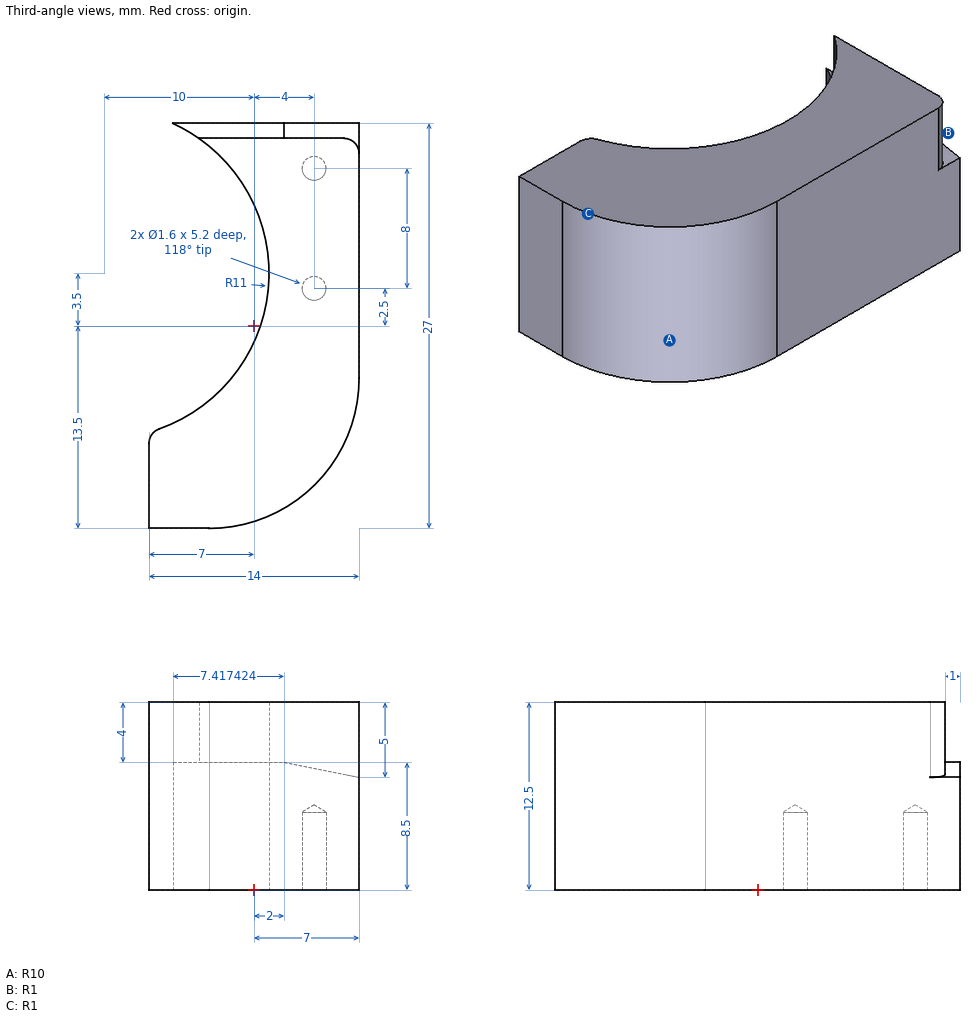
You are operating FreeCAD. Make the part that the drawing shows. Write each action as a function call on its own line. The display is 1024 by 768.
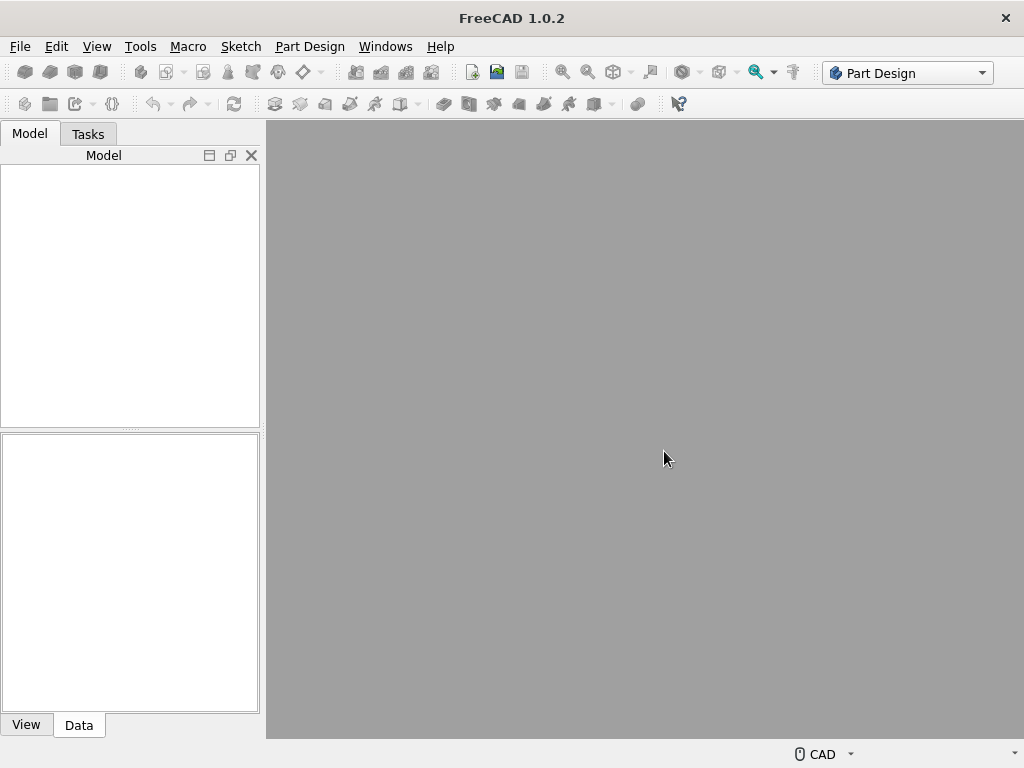
click(472, 72)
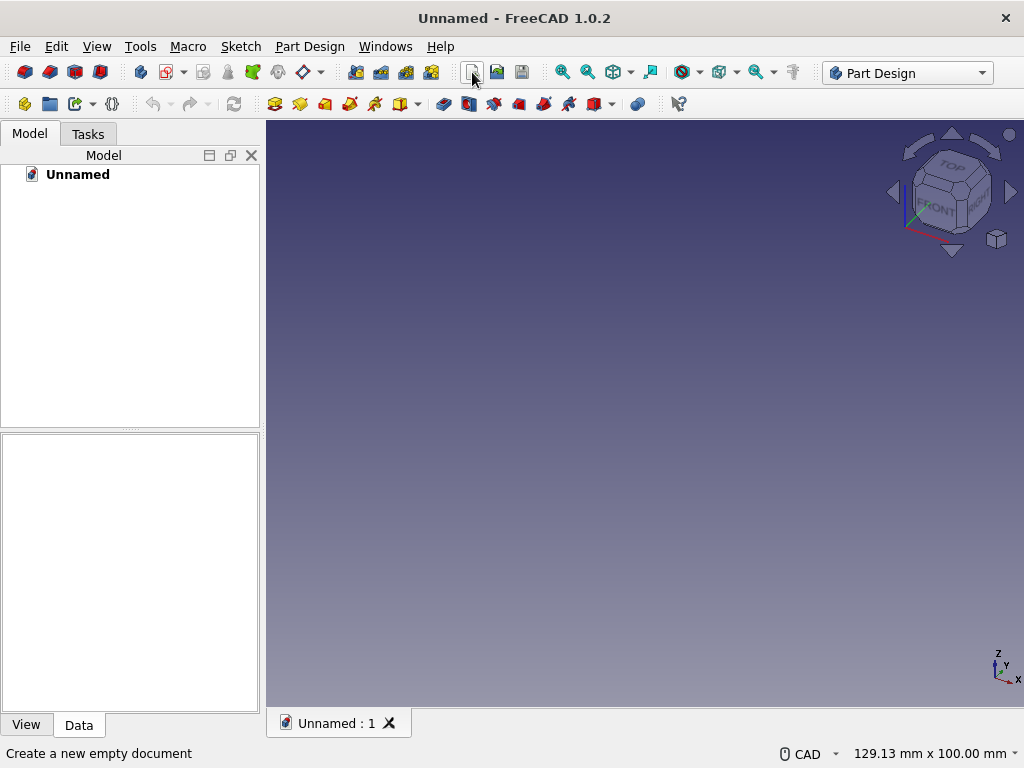
click(166, 72)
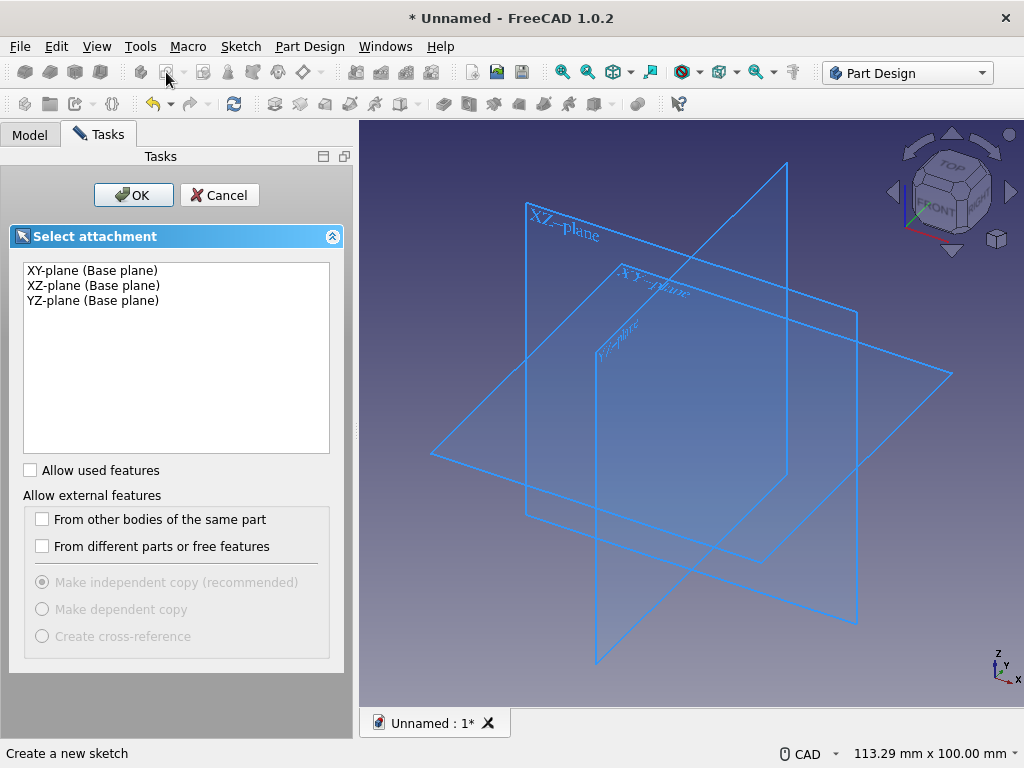
click(84, 270)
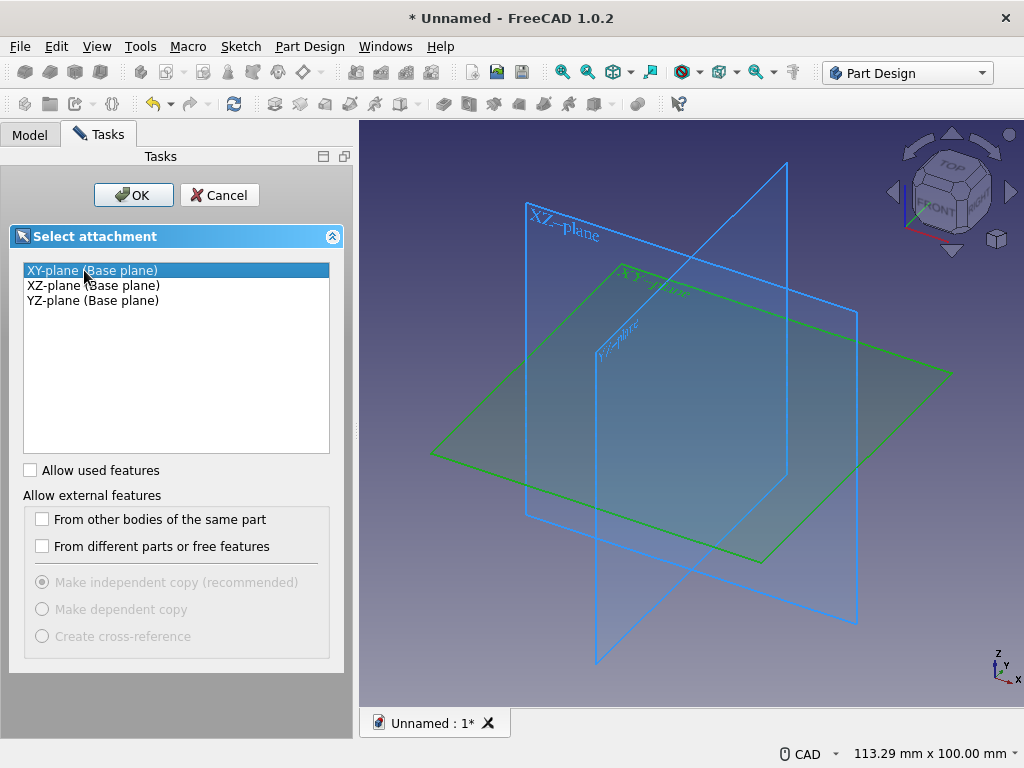
click(134, 195)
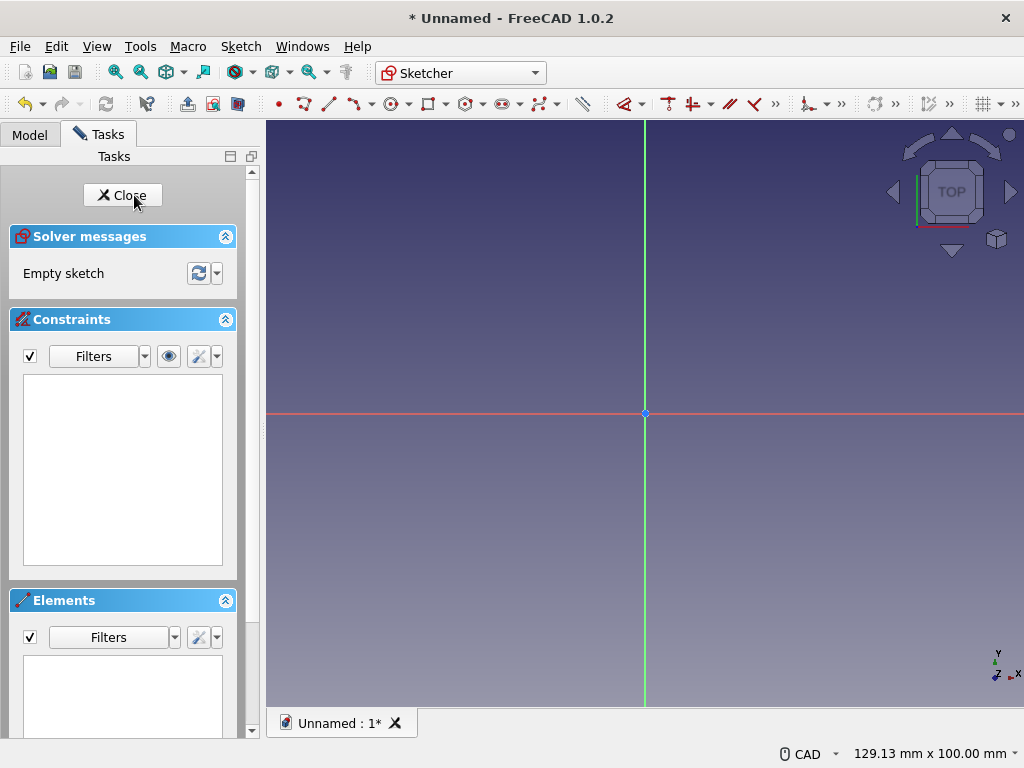
scroll(701, 413, up, 4)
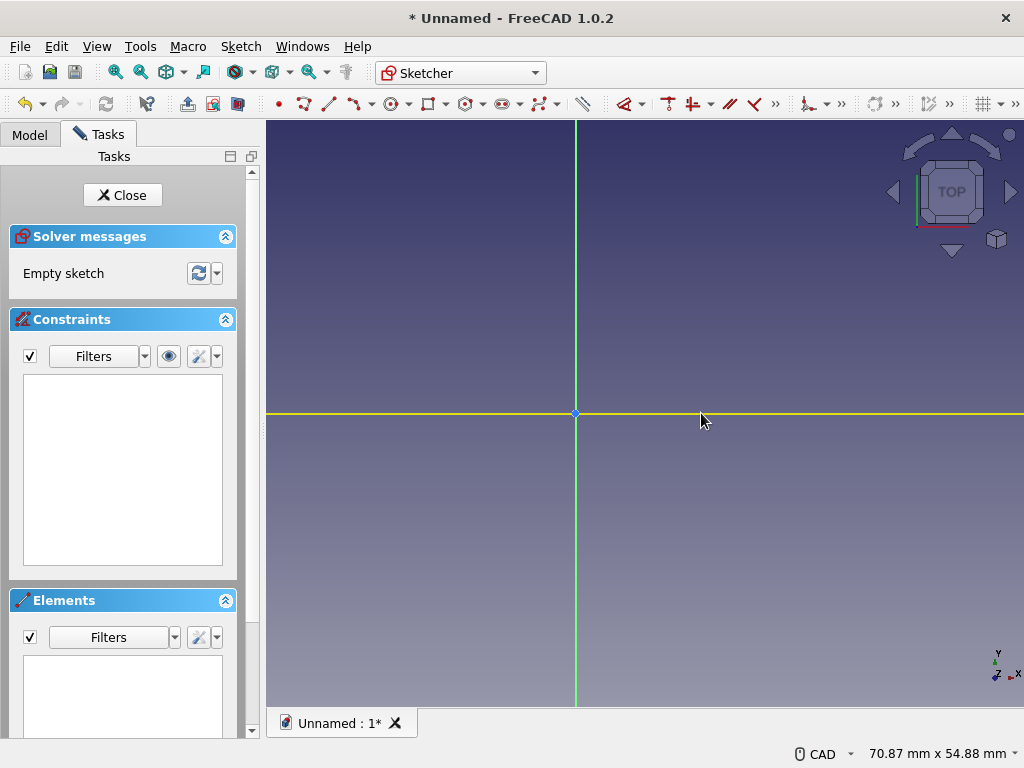
click(304, 104)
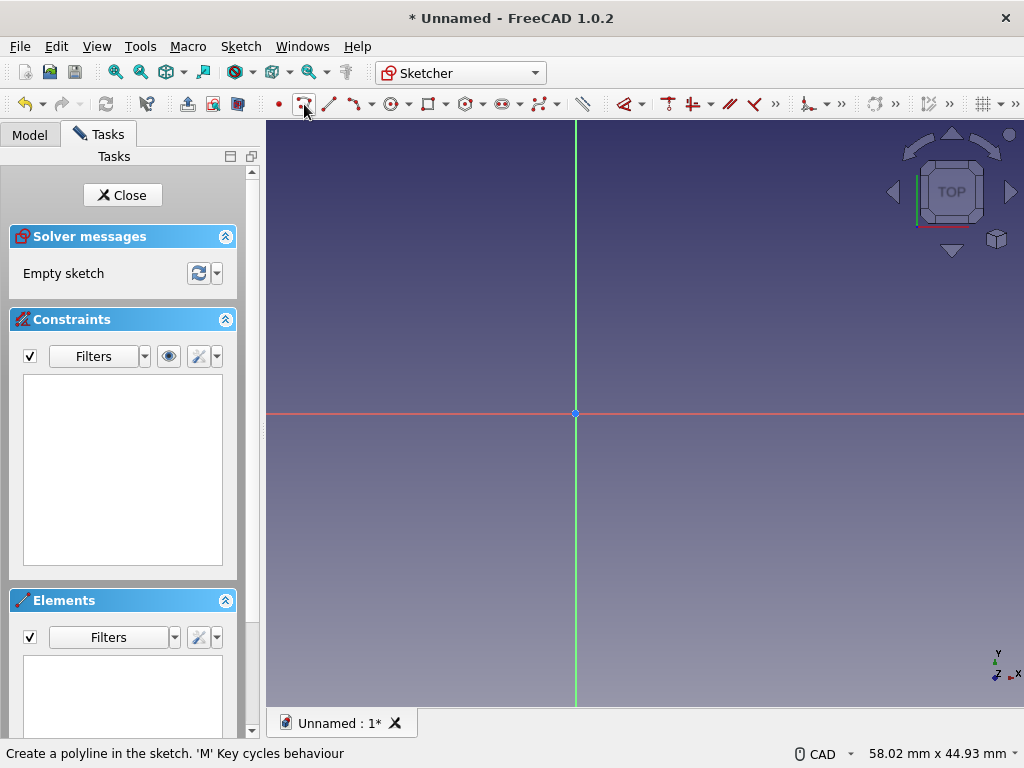
click(484, 506)
click(484, 590)
click(667, 590)
click(667, 237)
click(505, 237)
right_click(505, 237)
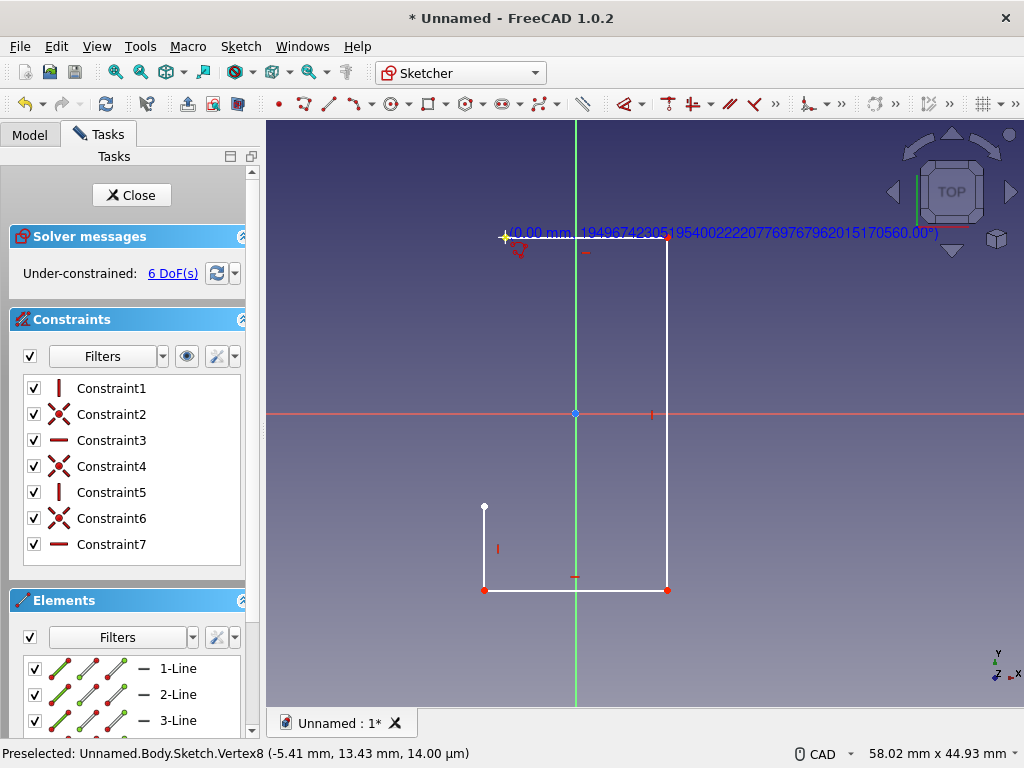
click(354, 104)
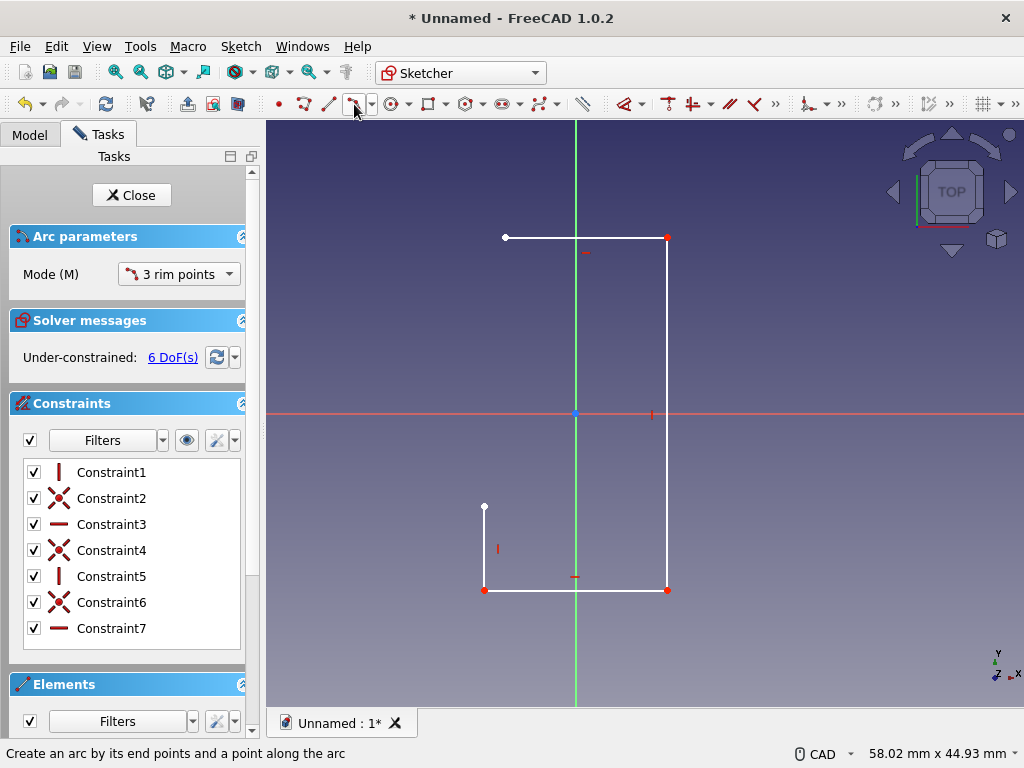
click(505, 238)
click(484, 507)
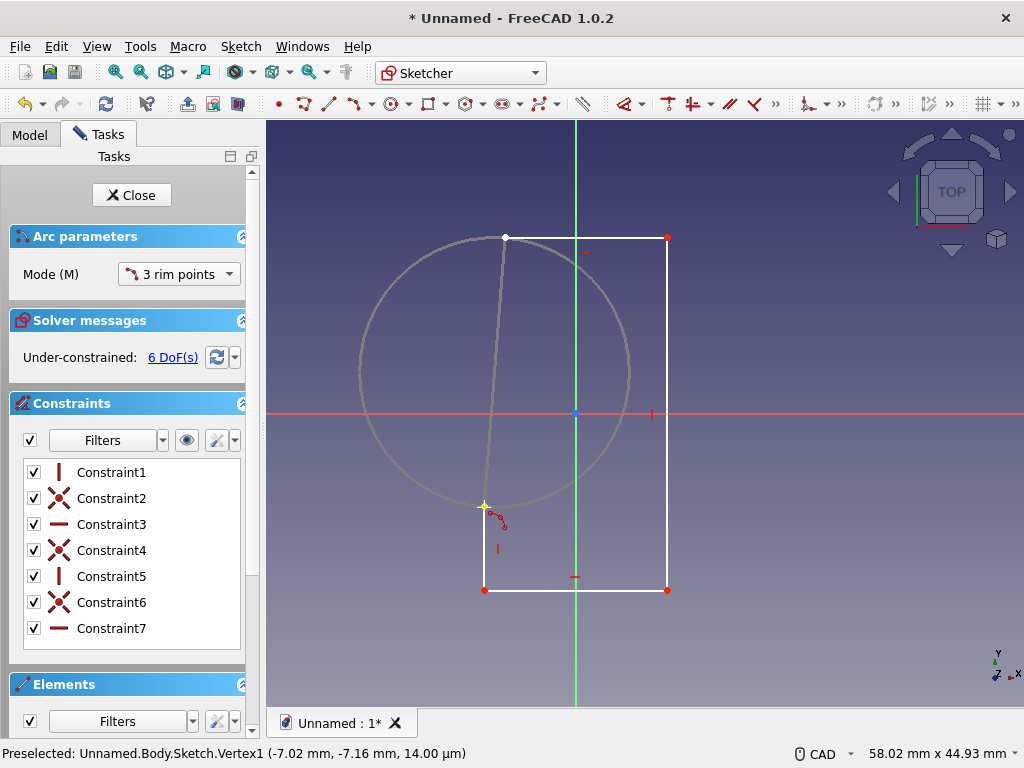
scroll(588, 379, up, 2)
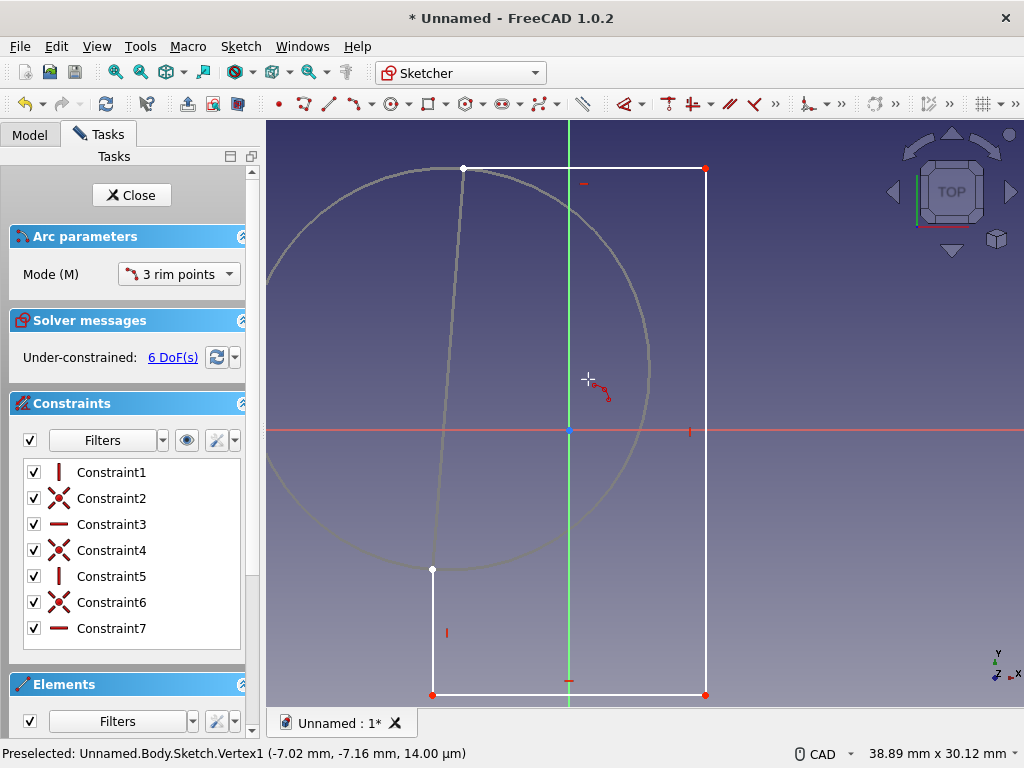
click(588, 378)
key(Escape)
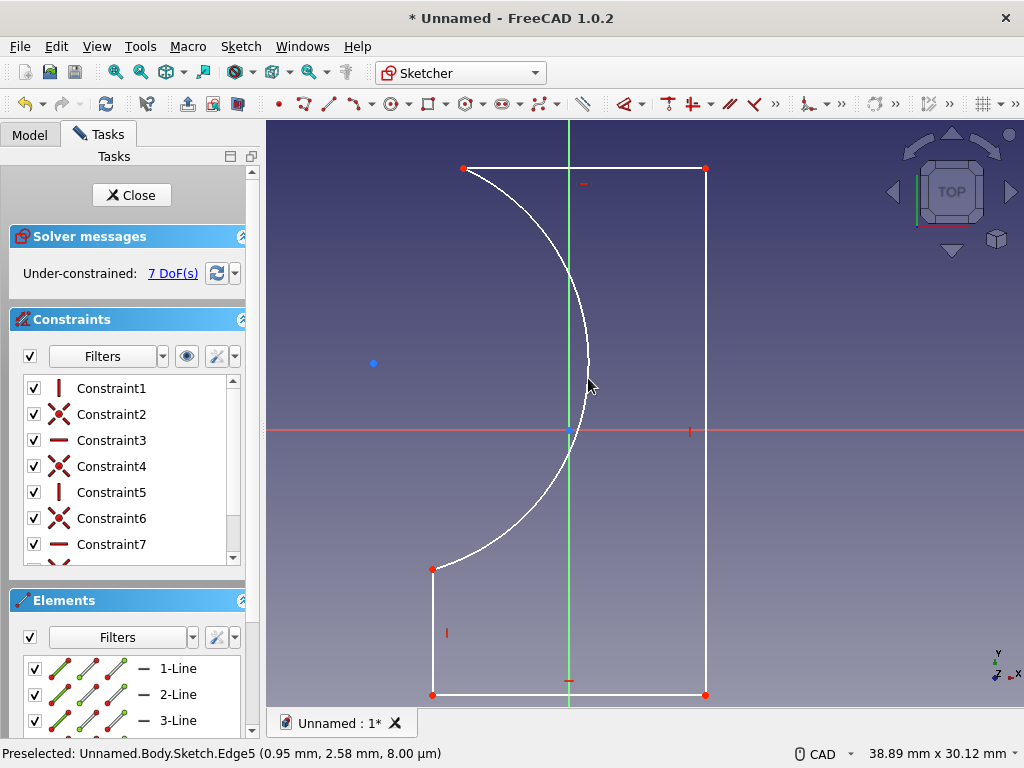
click(624, 104)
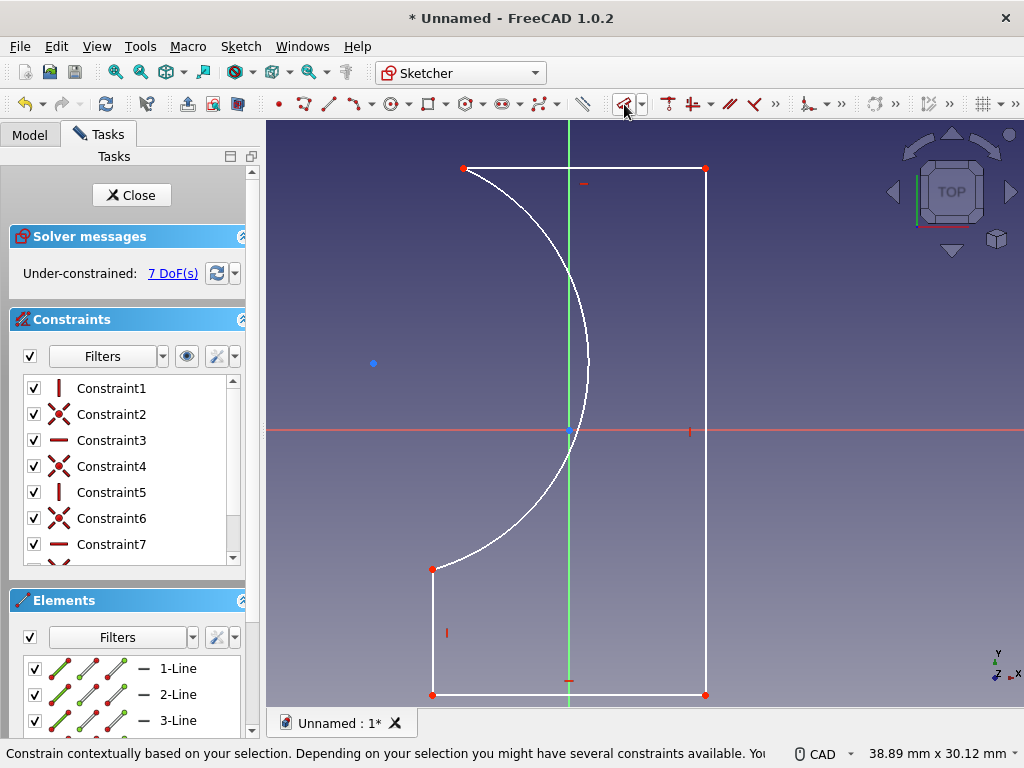
click(555, 478)
click(493, 579)